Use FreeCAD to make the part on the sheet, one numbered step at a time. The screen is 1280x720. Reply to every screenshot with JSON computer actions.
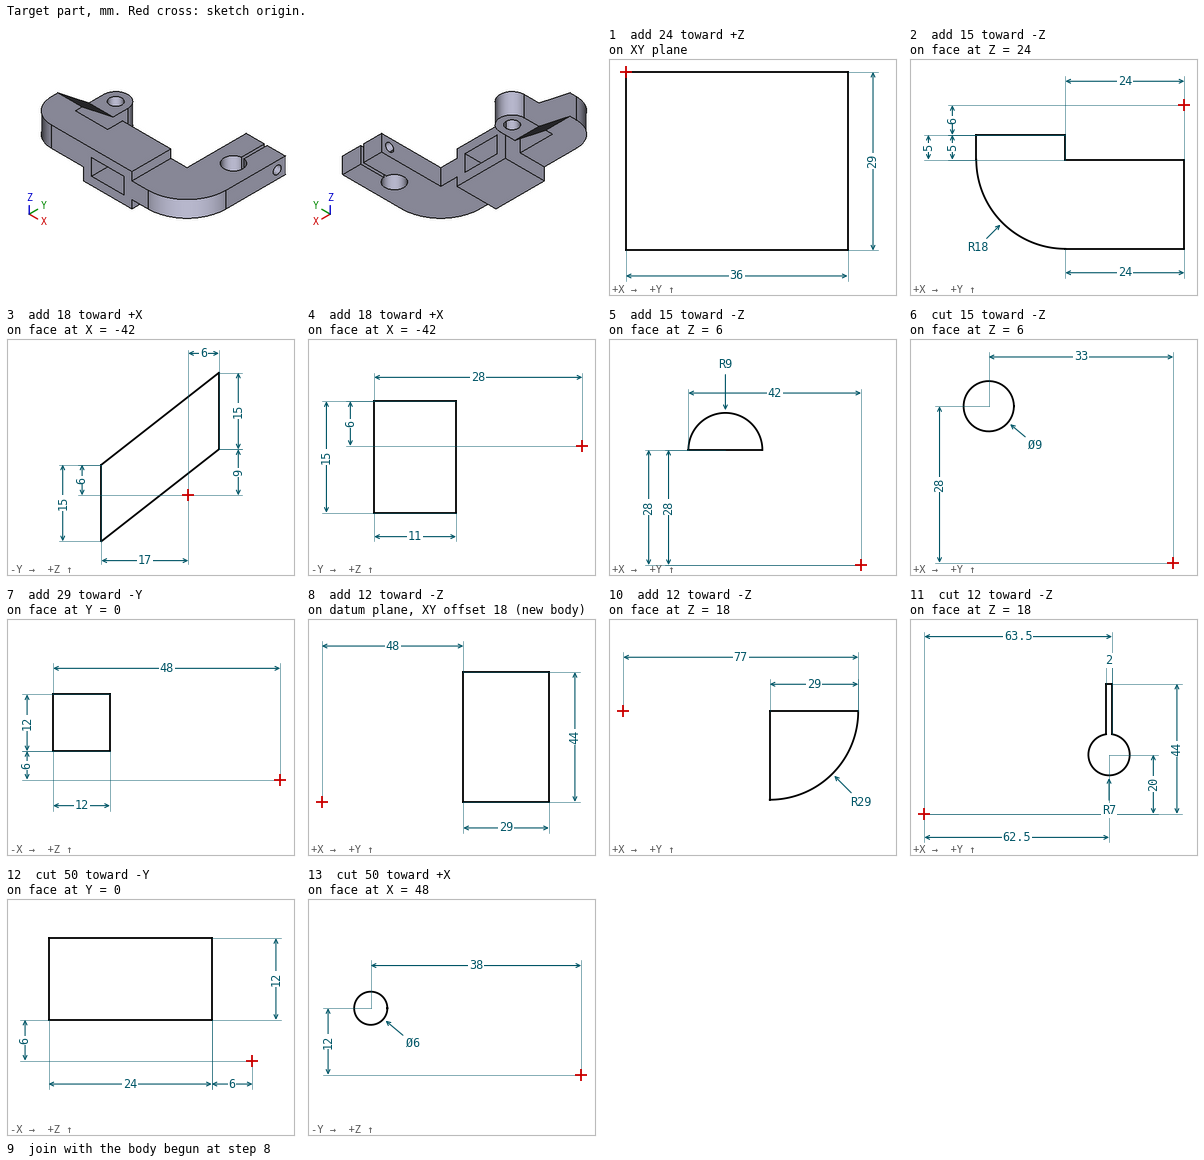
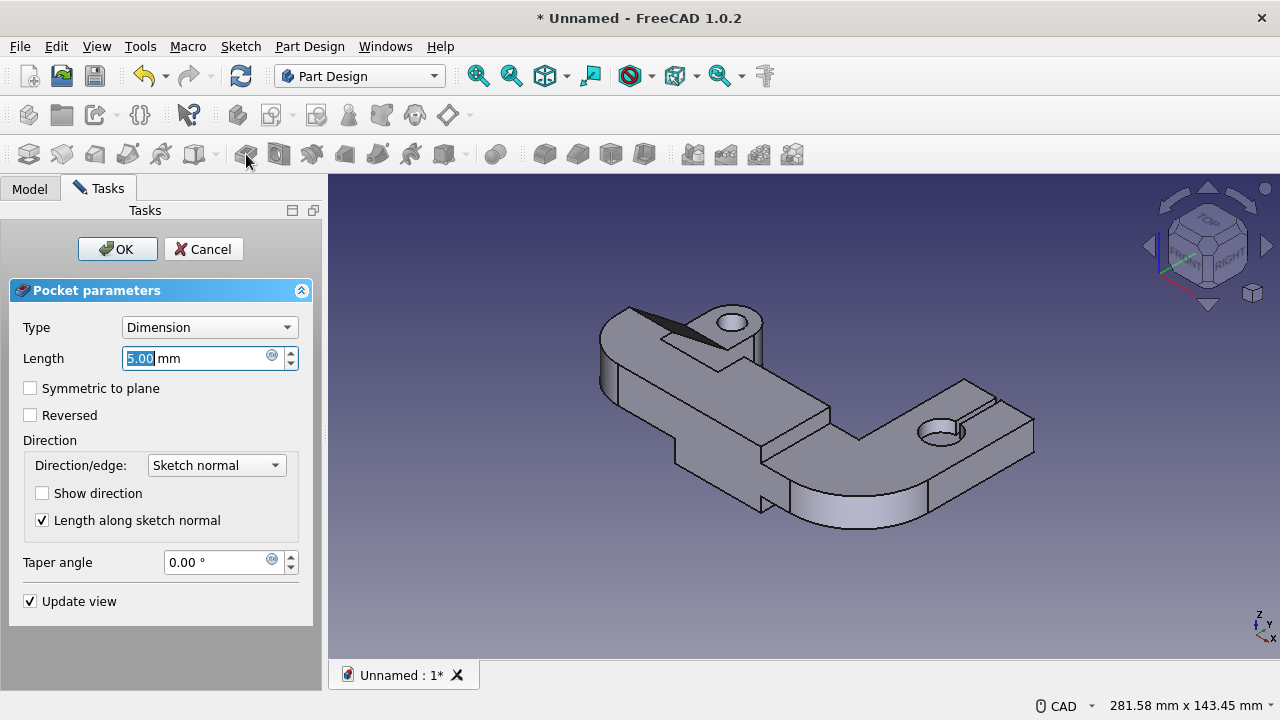
{"action": "type", "text": "12"}
{"action": "key", "text": "Tab"}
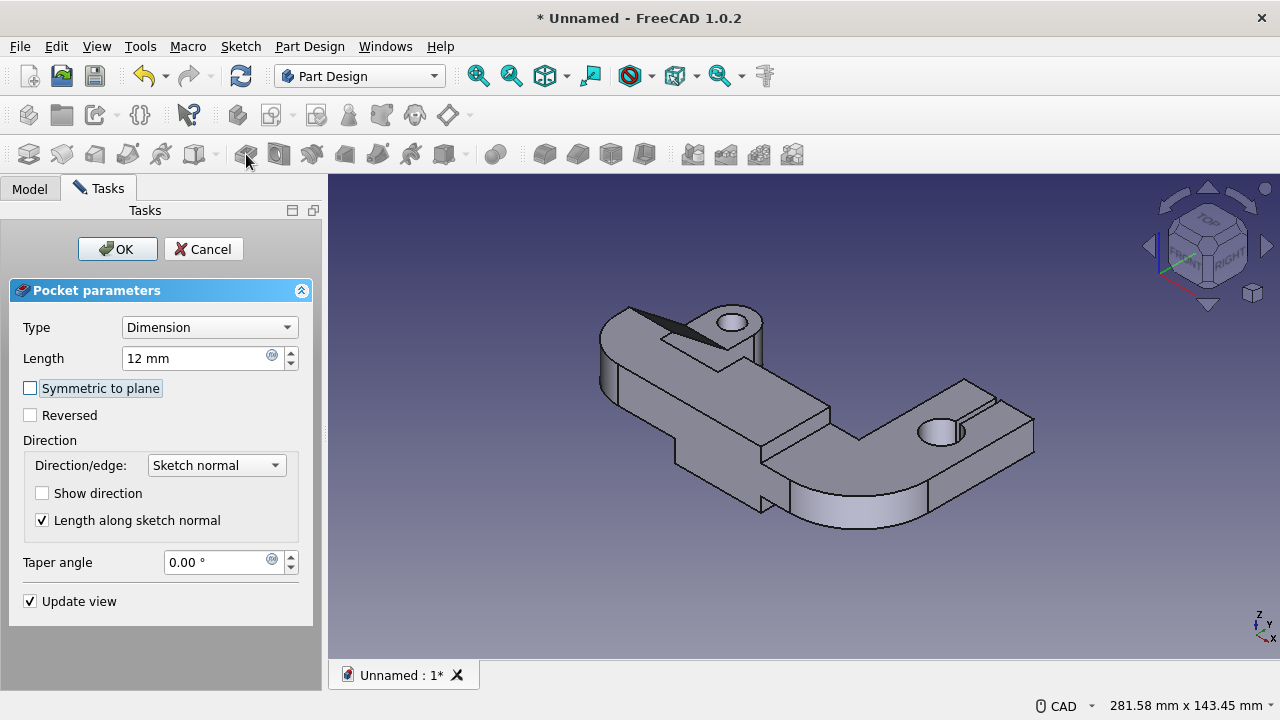
{"action": "left_click", "coordinate": [118, 249]}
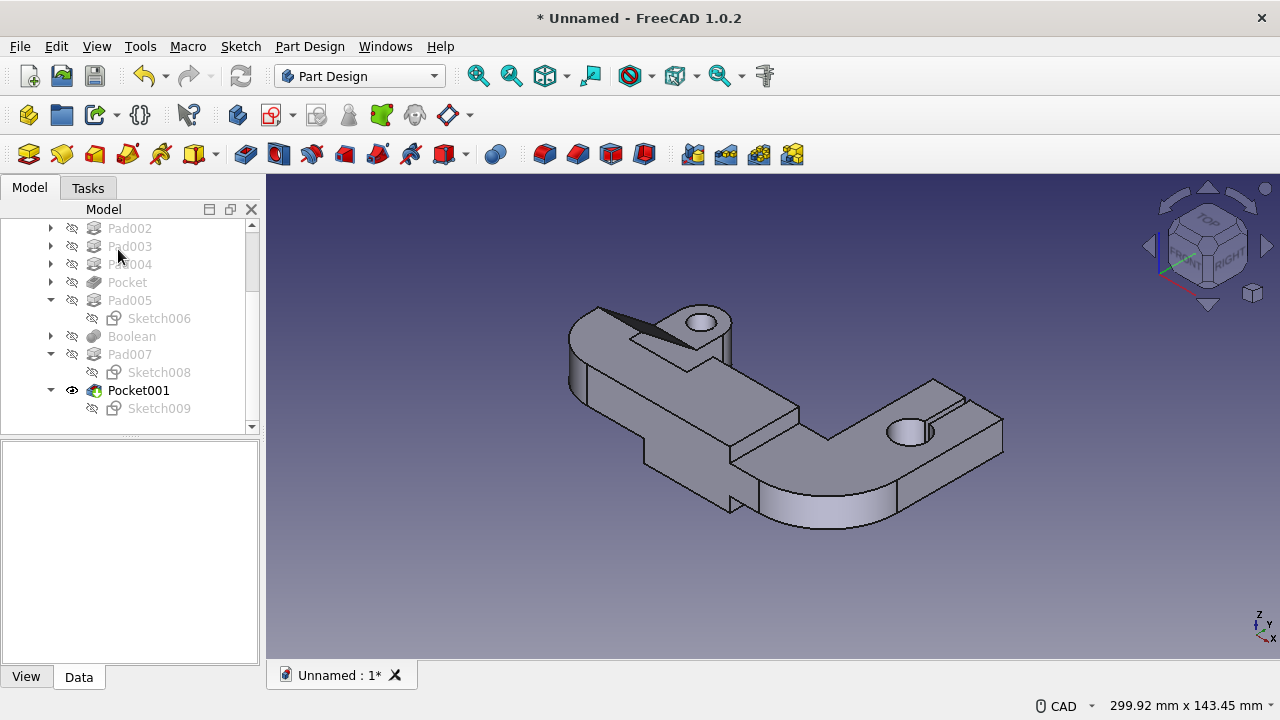
{"action": "key", "text": "4"}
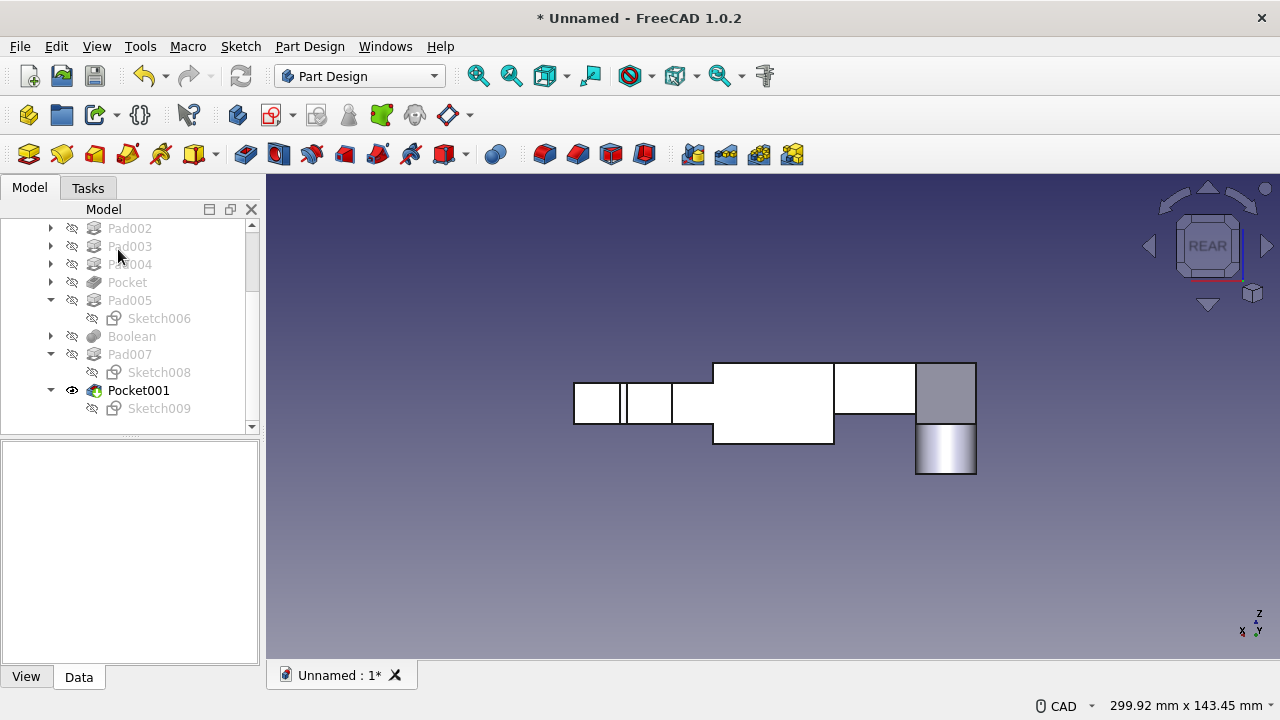
{"action": "key", "text": "v f"}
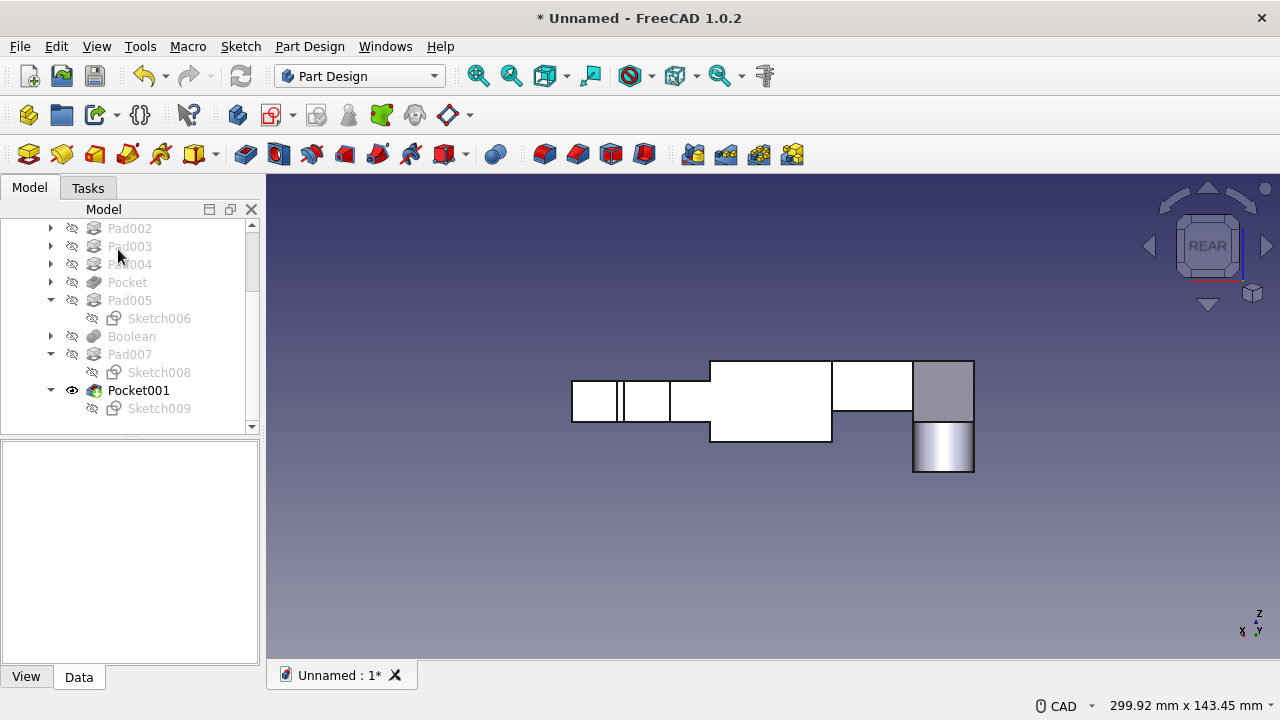
{"action": "left_click", "coordinate": [751, 400]}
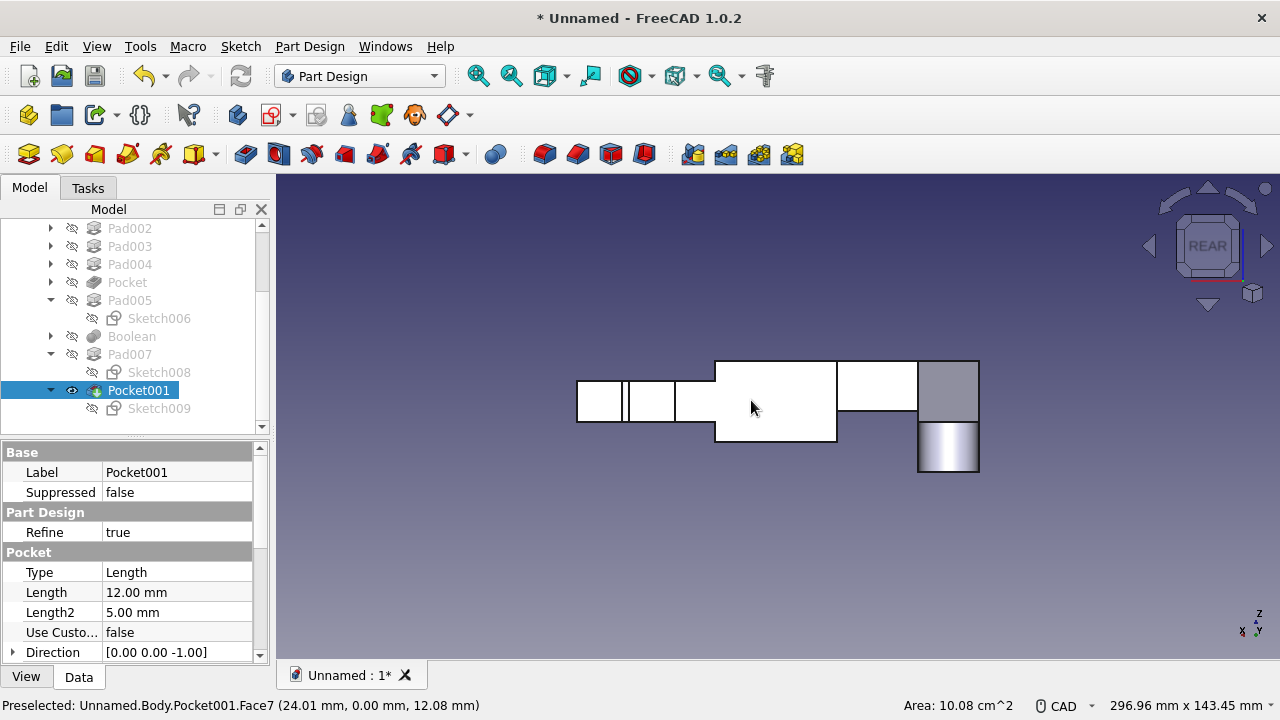
{"action": "left_click", "coordinate": [270, 116]}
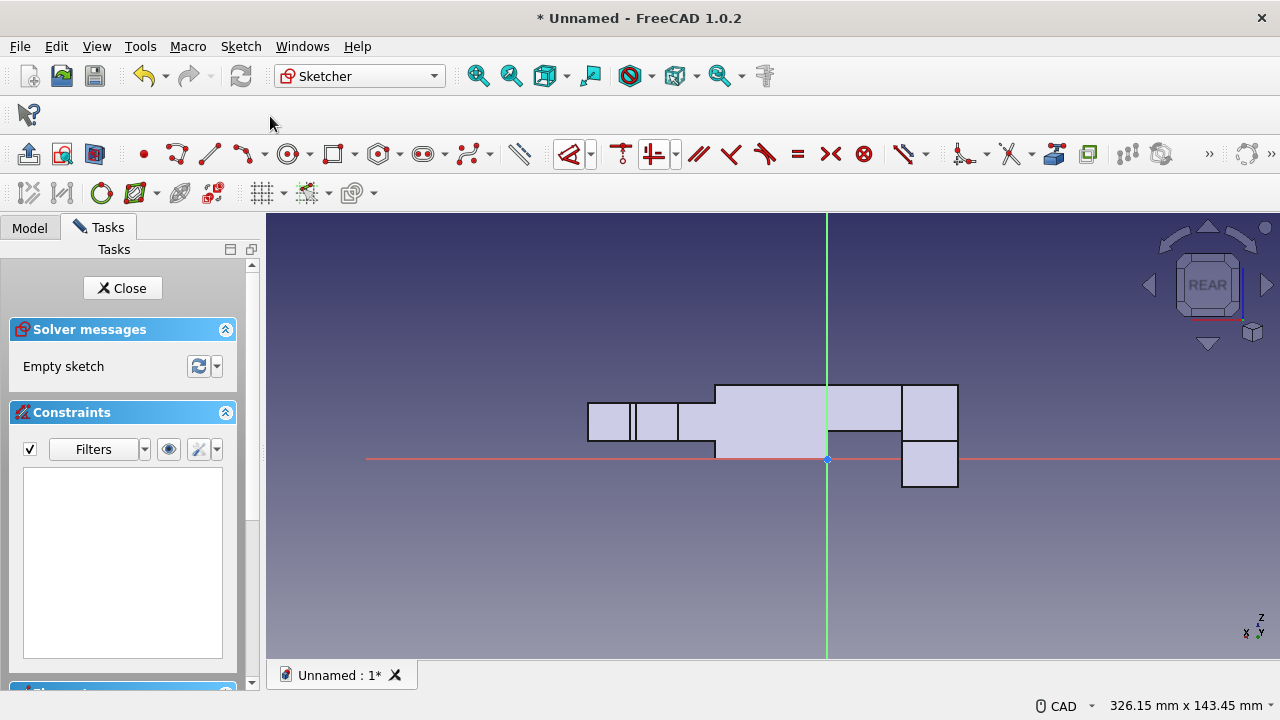
{"action": "scroll", "coordinate": [800, 430], "scroll_direction": "up", "scroll_amount": 8}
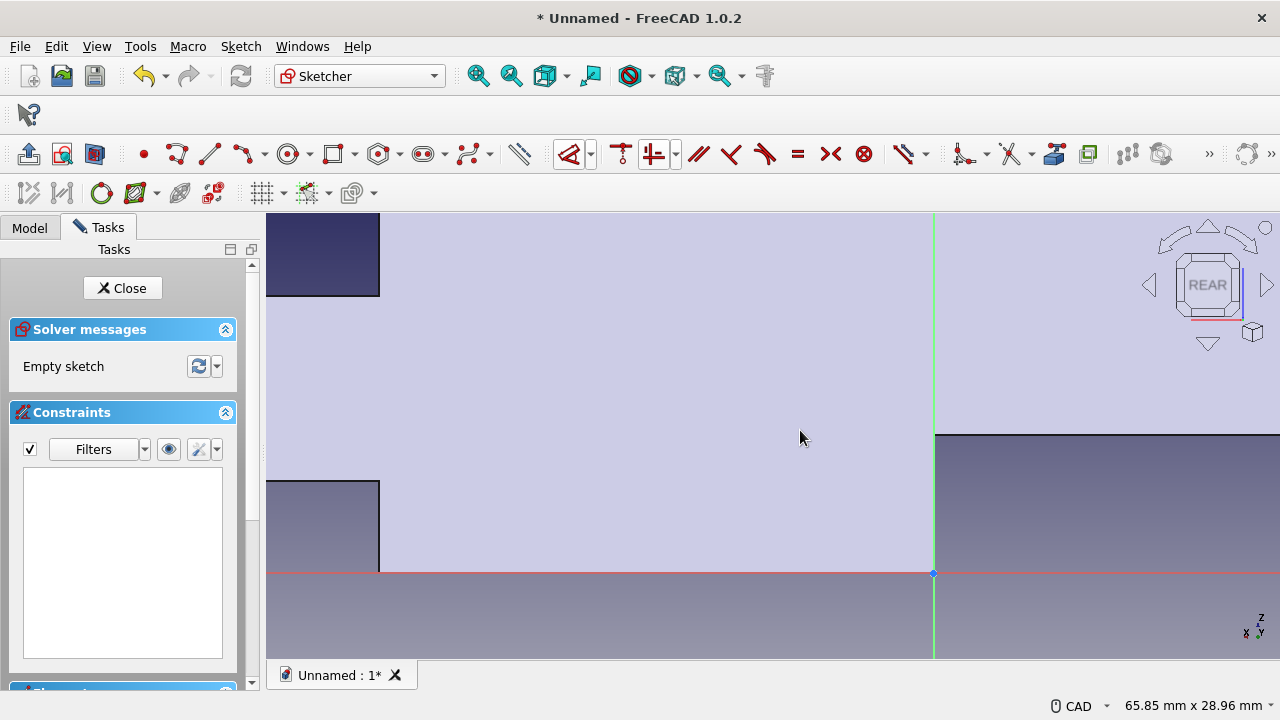
{"action": "key", "text": "g r"}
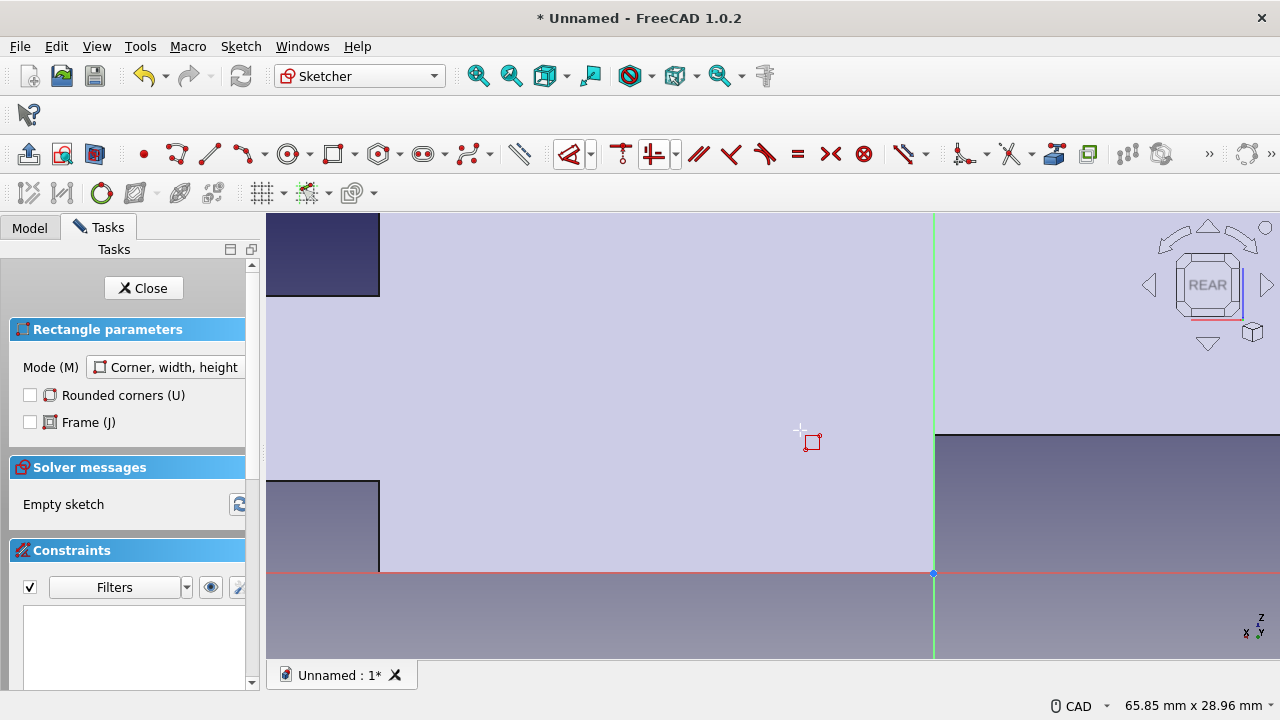
{"action": "left_click", "coordinate": [472, 296]}
{"action": "mouse_move", "coordinate": [841, 481]}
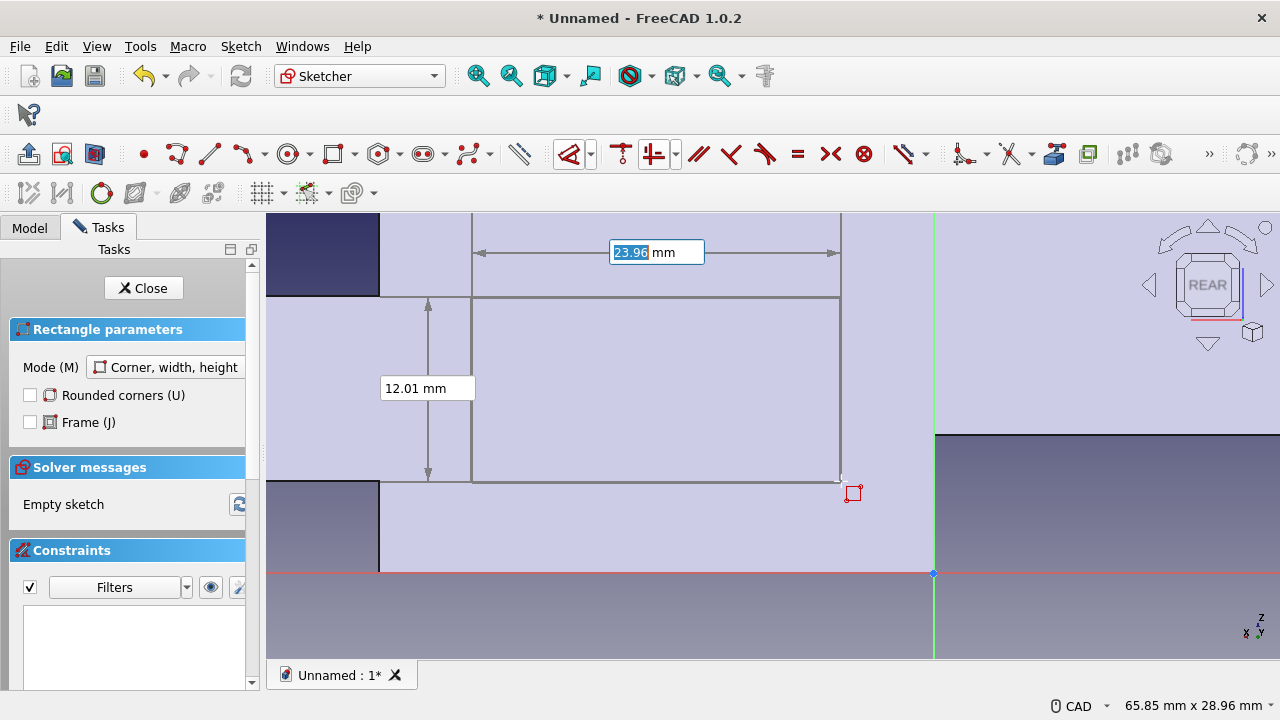
{"action": "type", "text": "24"}
{"action": "key", "text": "Tab"}
{"action": "type", "text": "12"}
{"action": "key", "text": "Return"}
{"action": "key", "text": "Escape"}